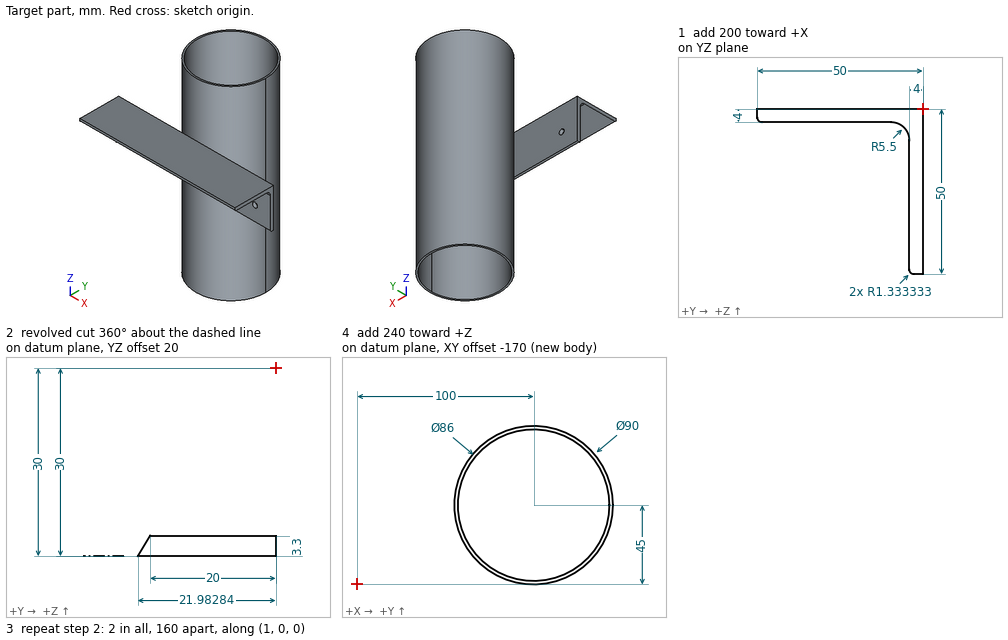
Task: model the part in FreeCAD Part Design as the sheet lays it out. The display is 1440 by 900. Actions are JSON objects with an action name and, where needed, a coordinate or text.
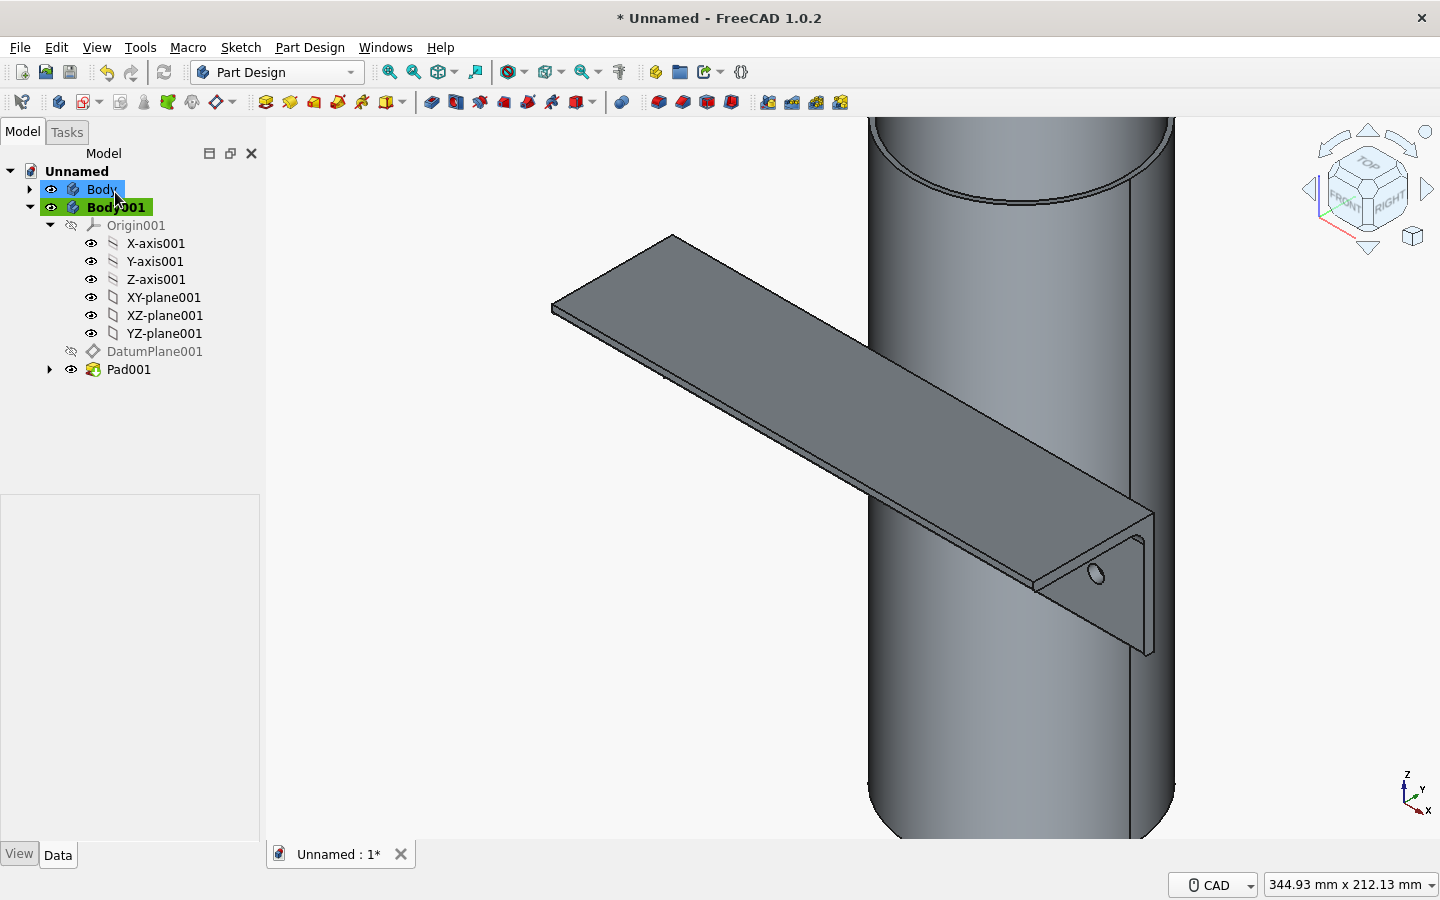
{"action": "left_click", "coordinate": [390, 72]}